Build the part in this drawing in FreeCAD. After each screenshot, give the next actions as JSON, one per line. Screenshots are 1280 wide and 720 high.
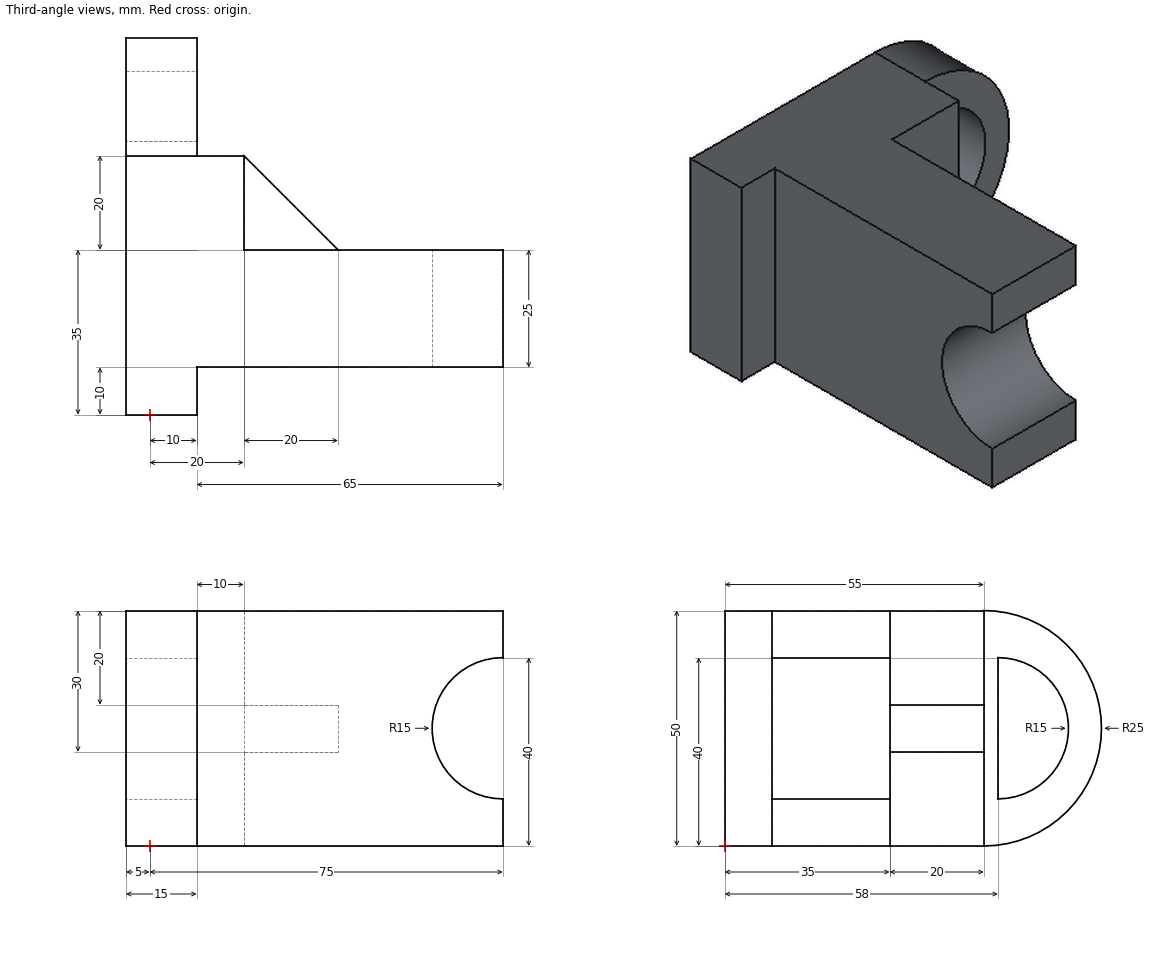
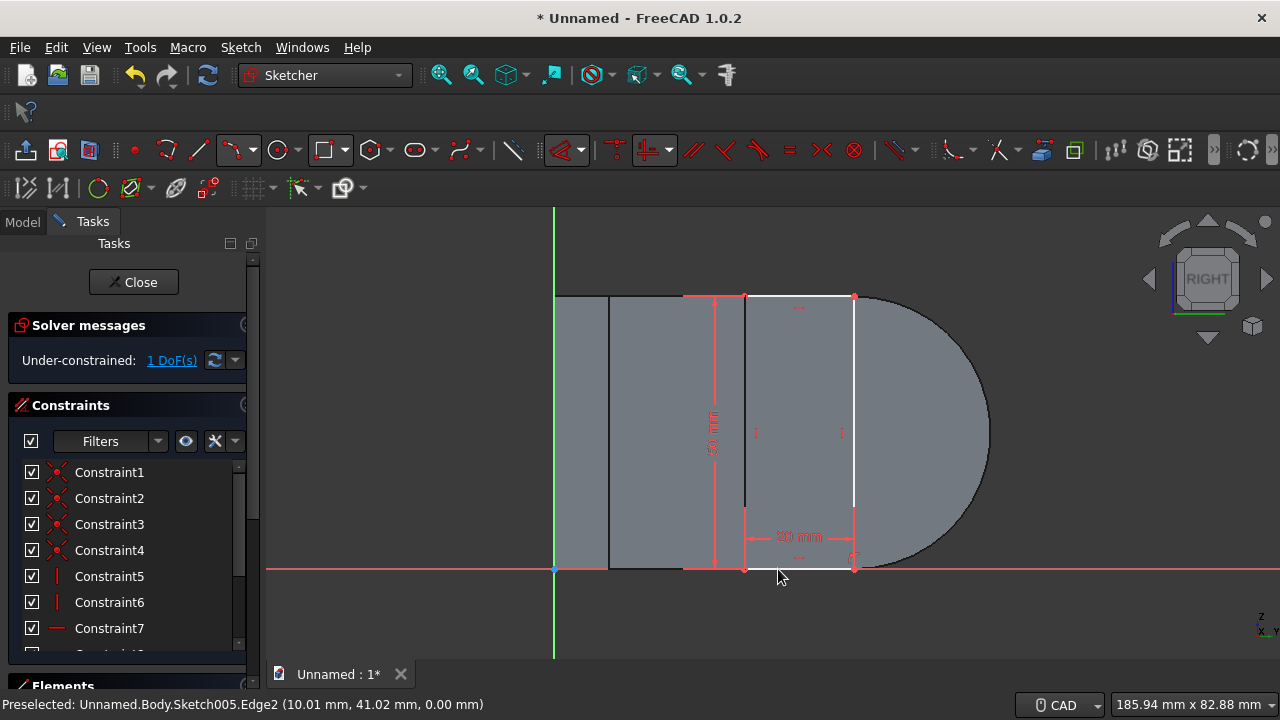
{"action": "left_click", "coordinate": [745, 296]}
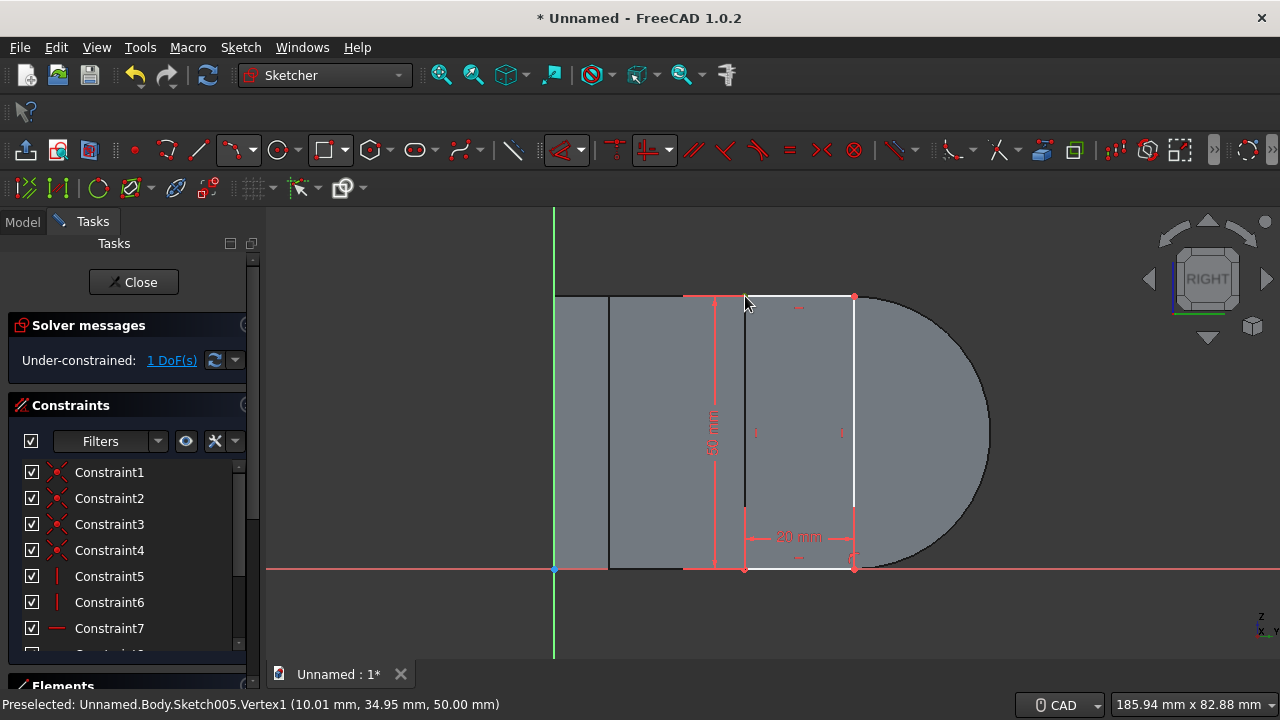
{"action": "left_click", "coordinate": [584, 150]}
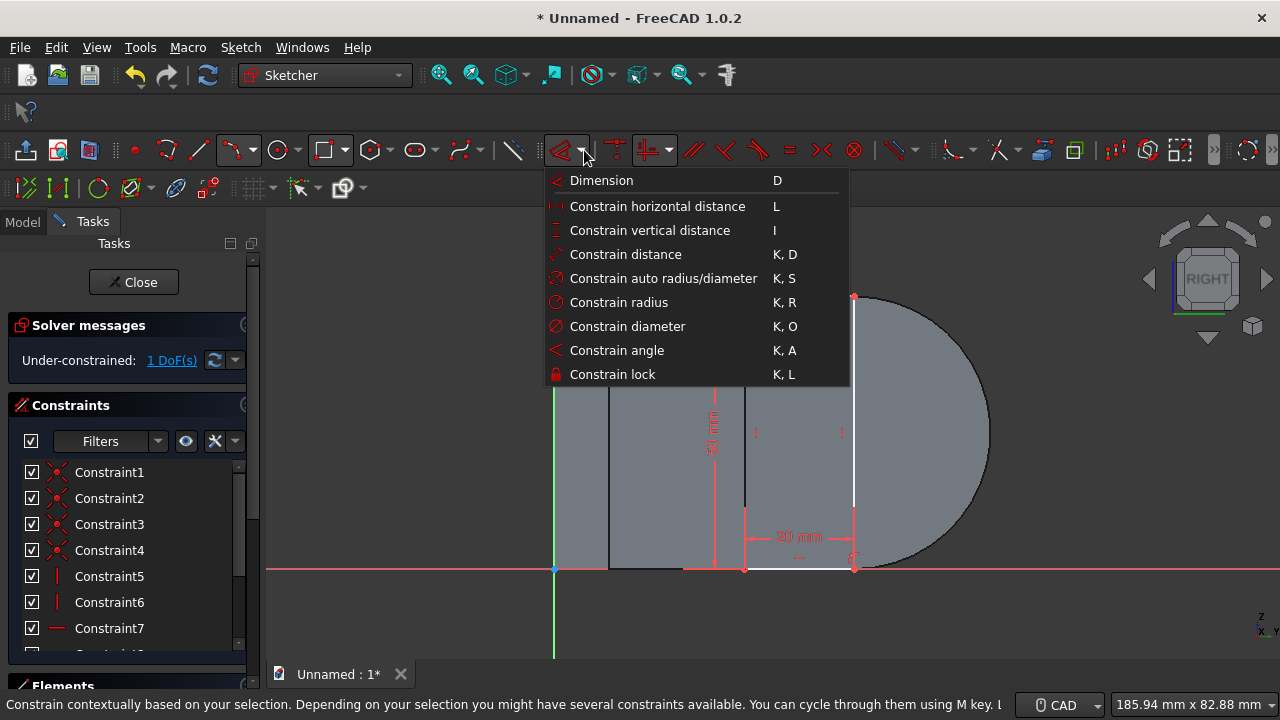
{"action": "left_click", "coordinate": [697, 206]}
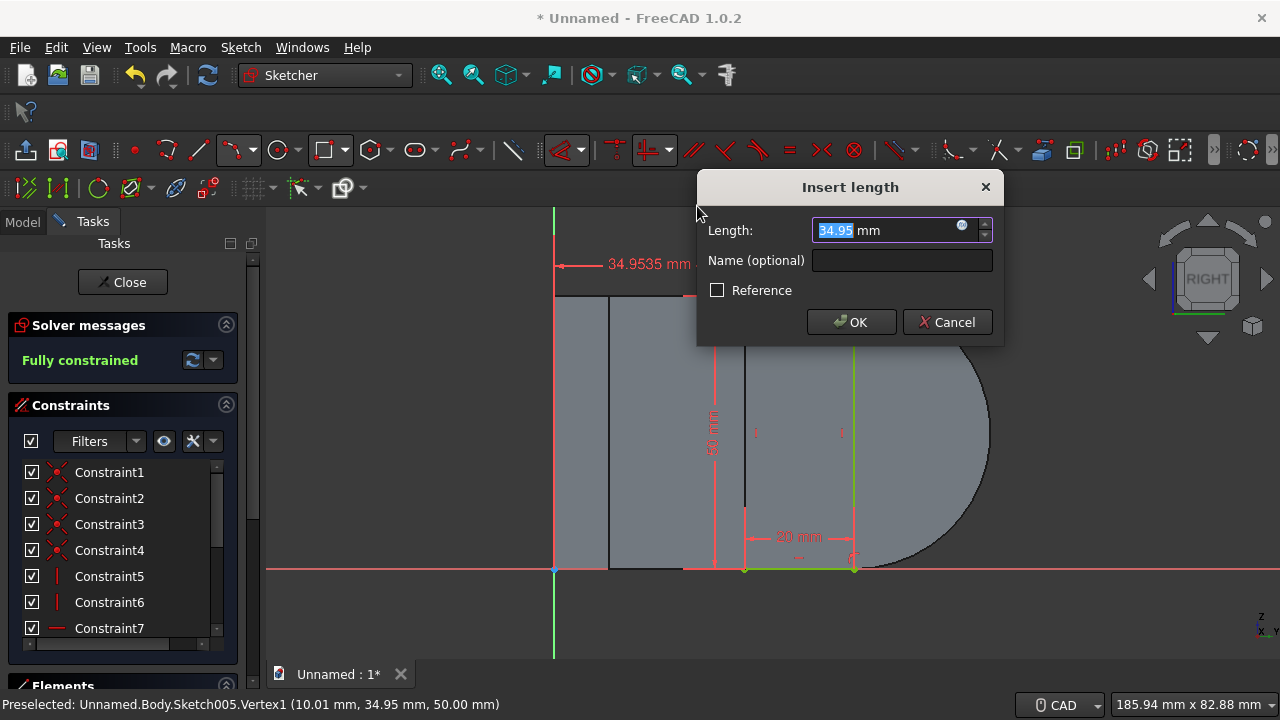
{"action": "type", "text": "35"}
{"action": "key", "text": "Return"}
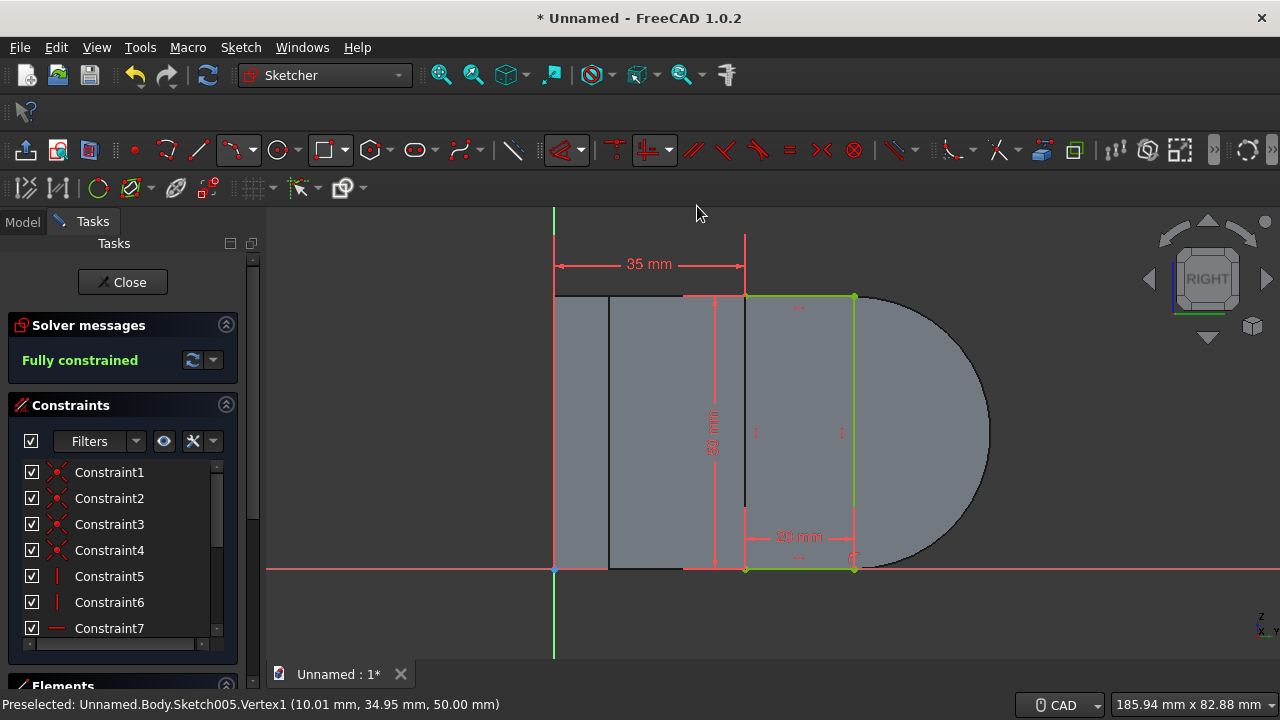
{"action": "left_click", "coordinate": [123, 282]}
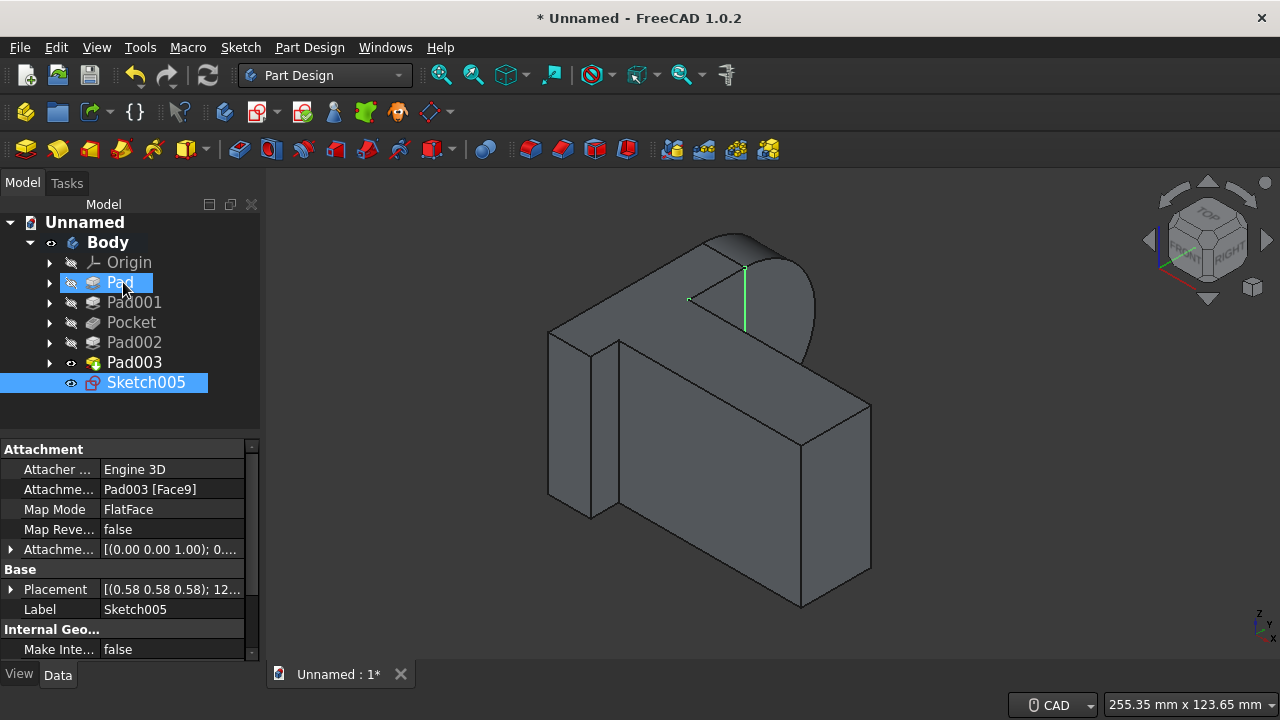
{"action": "left_click", "coordinate": [26, 150]}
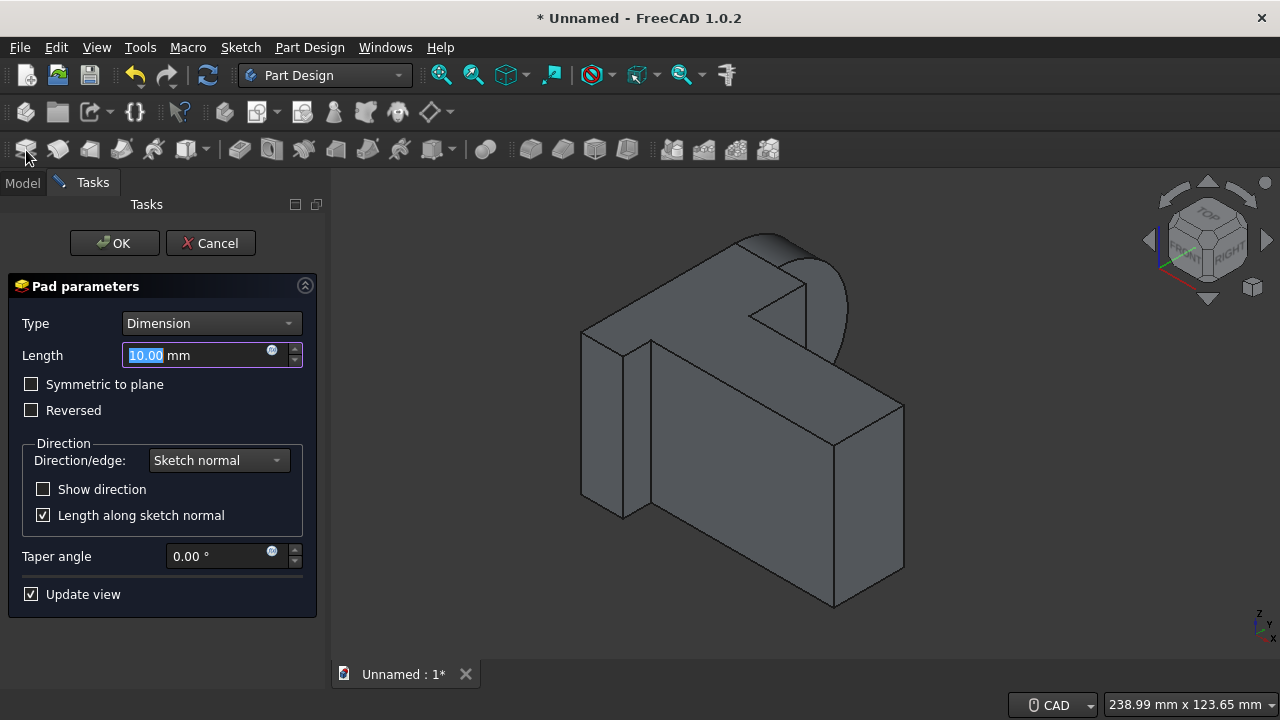
{"action": "type", "text": "10"}
{"action": "key", "text": "Tab"}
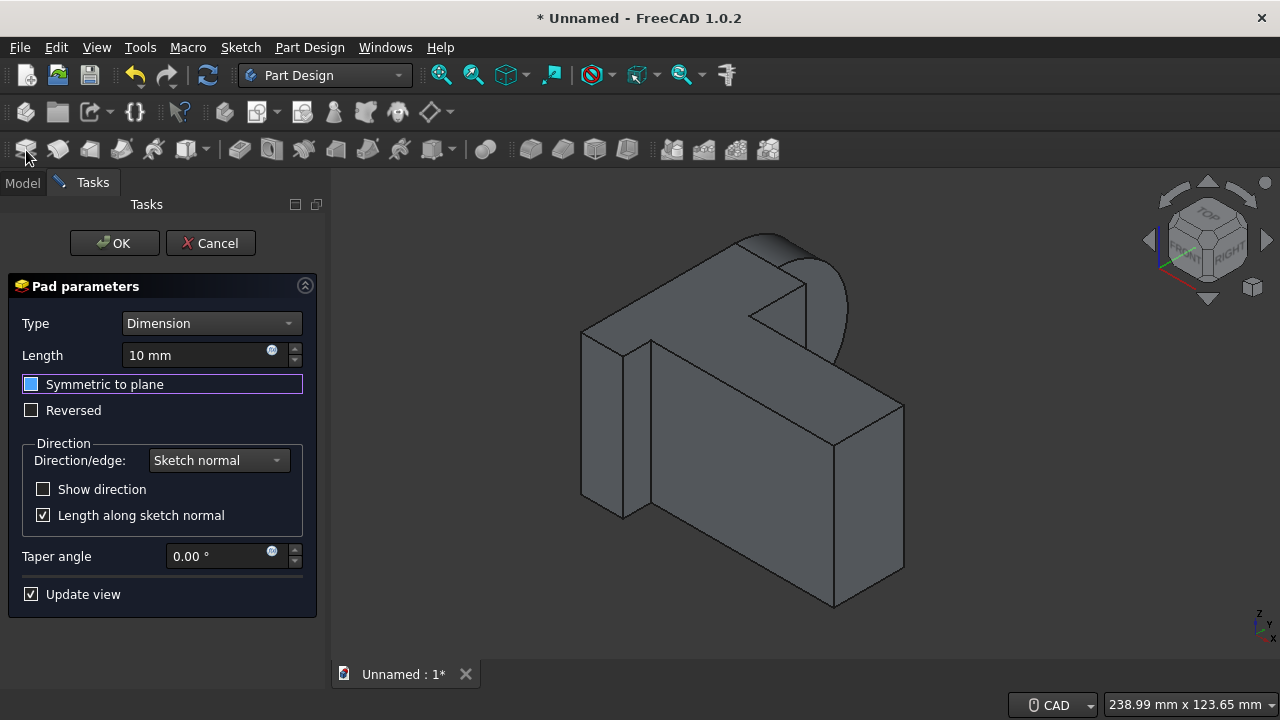
{"action": "left_click", "coordinate": [115, 243]}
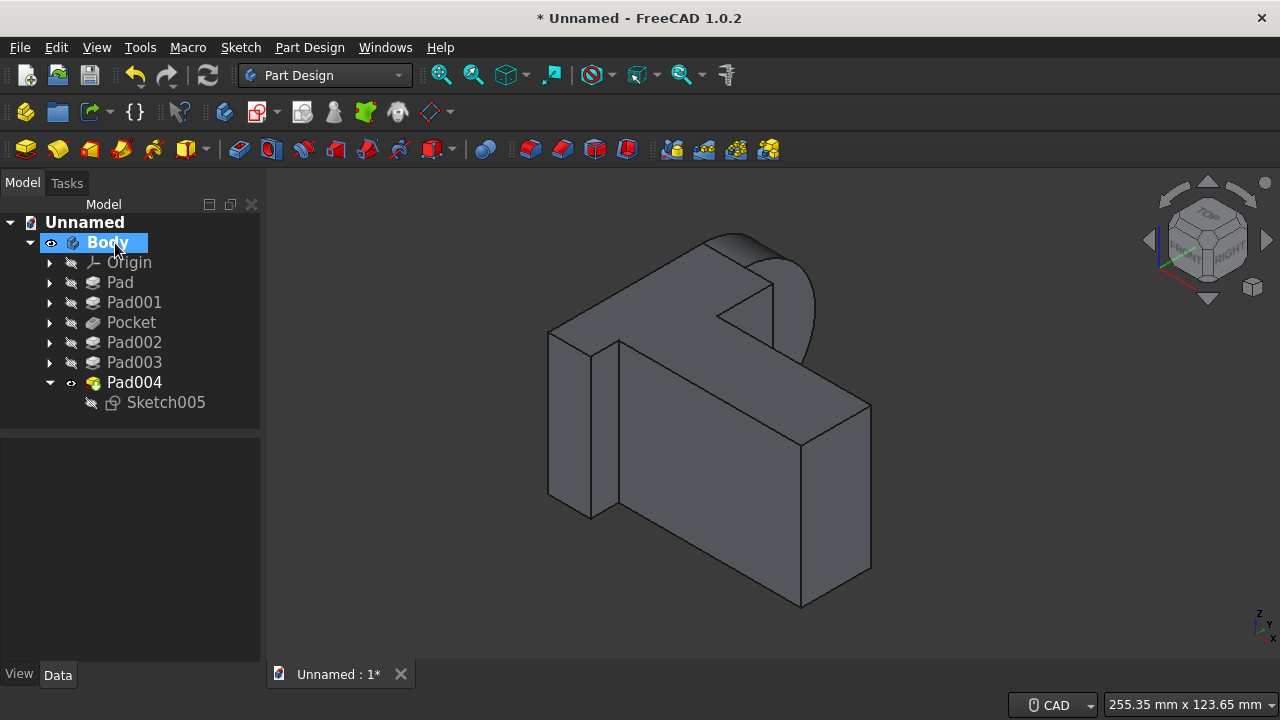
{"action": "left_click", "coordinate": [790, 322]}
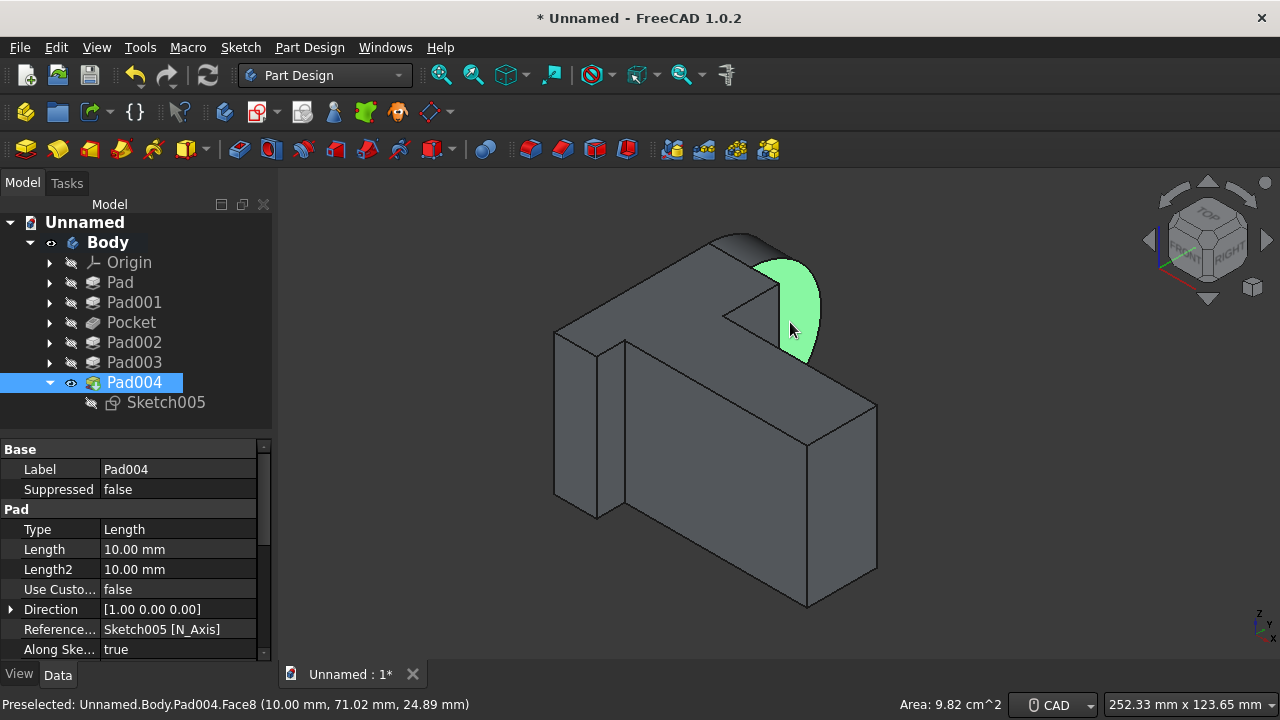
{"action": "left_click", "coordinate": [258, 112]}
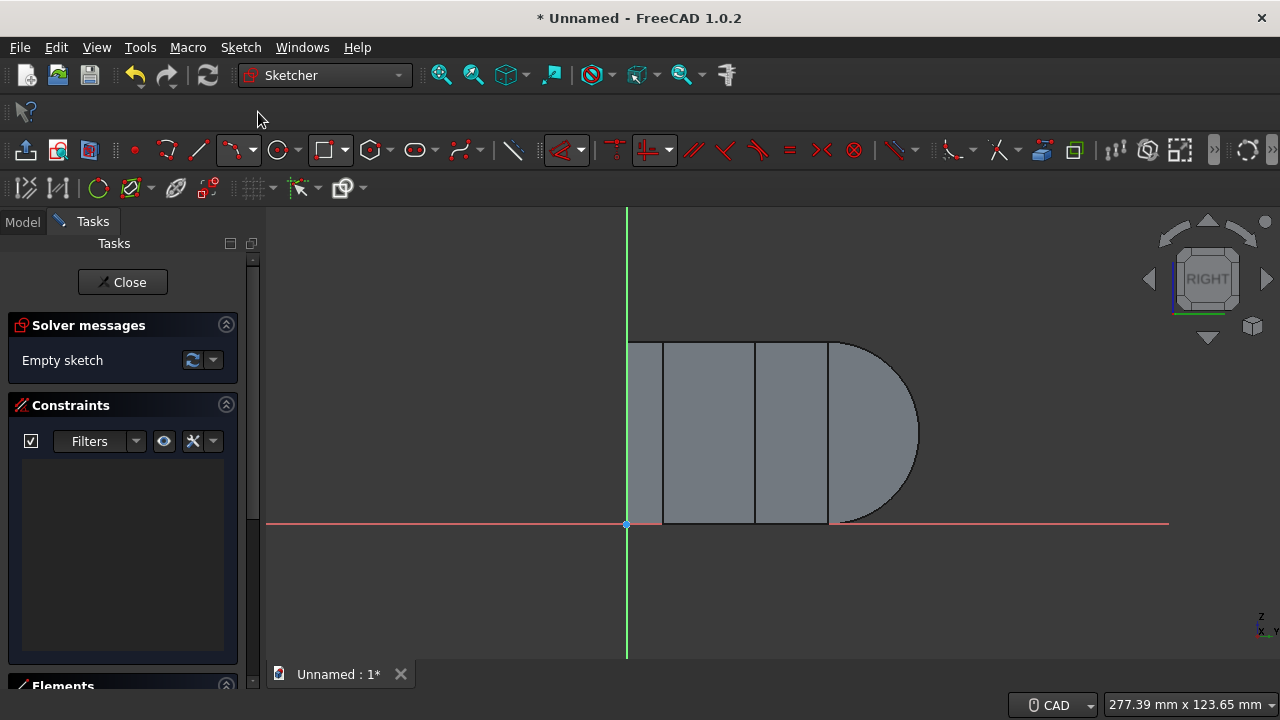
{"action": "left_click", "coordinate": [90, 150]}